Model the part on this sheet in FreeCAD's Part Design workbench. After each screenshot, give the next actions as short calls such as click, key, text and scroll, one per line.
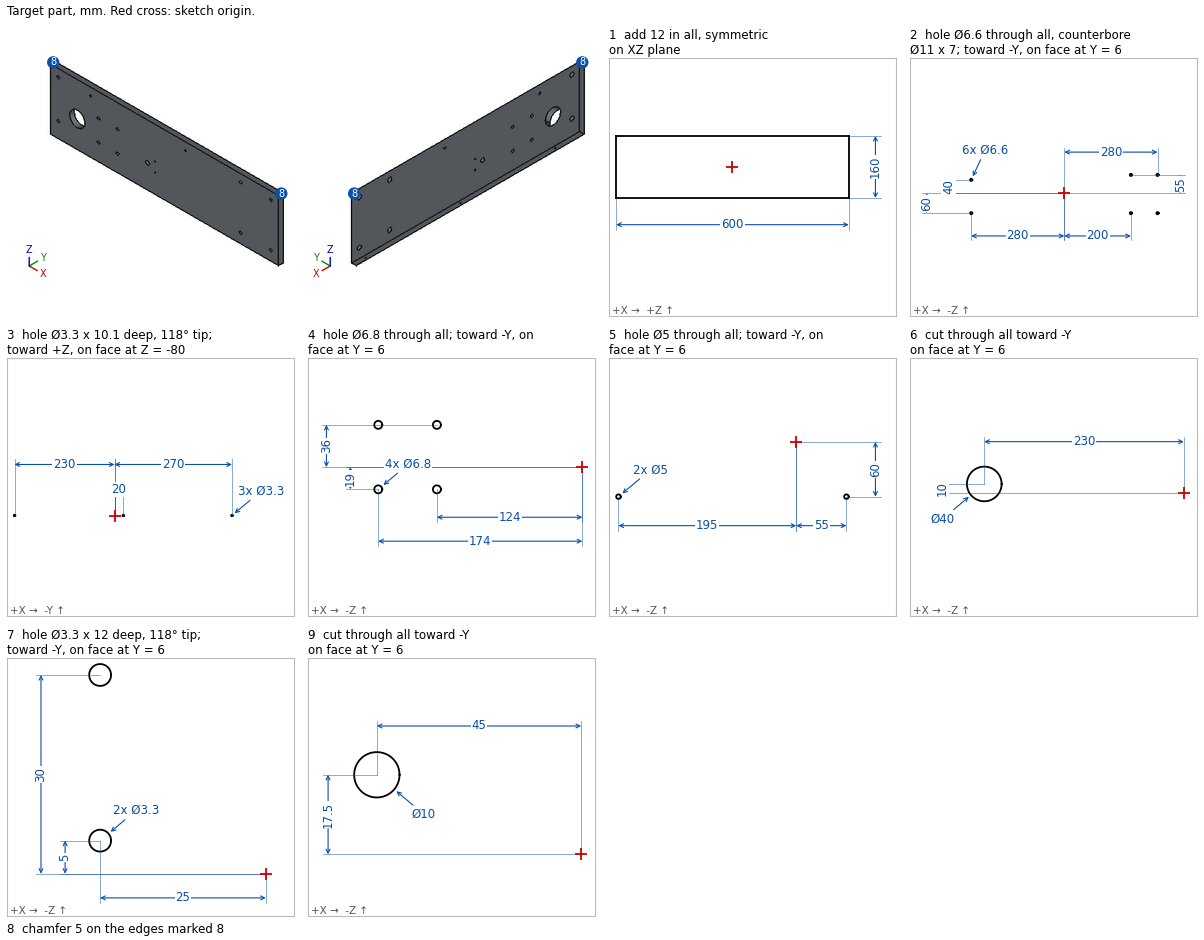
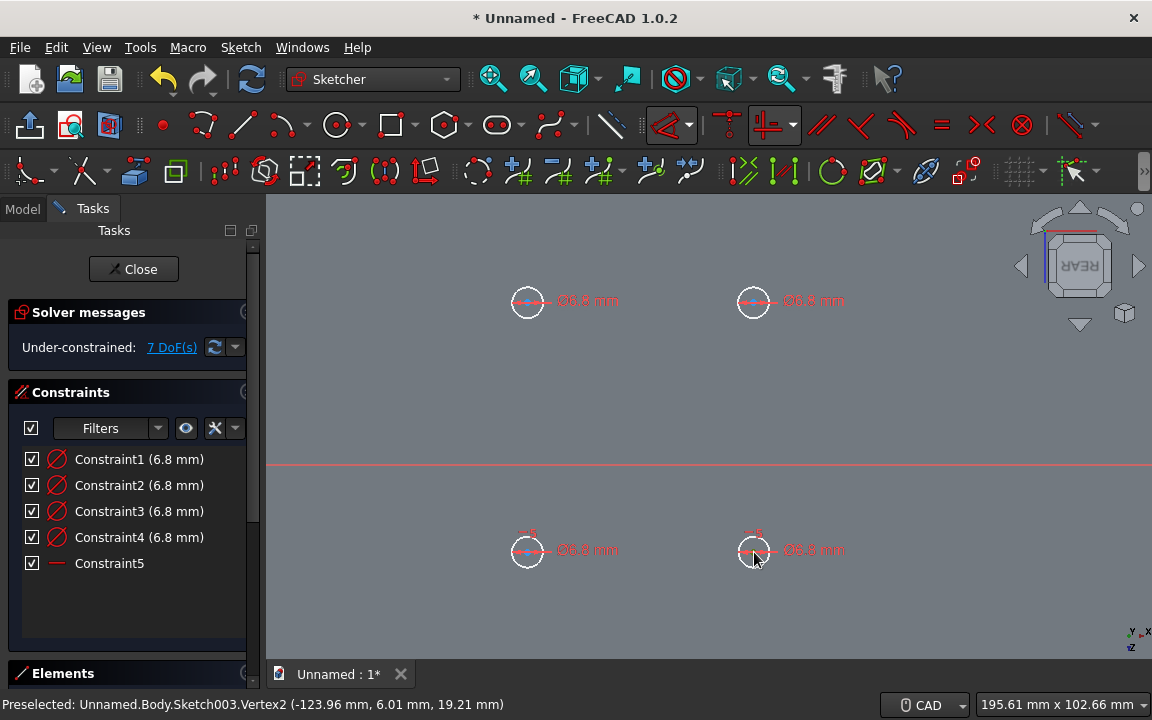
click(754, 303)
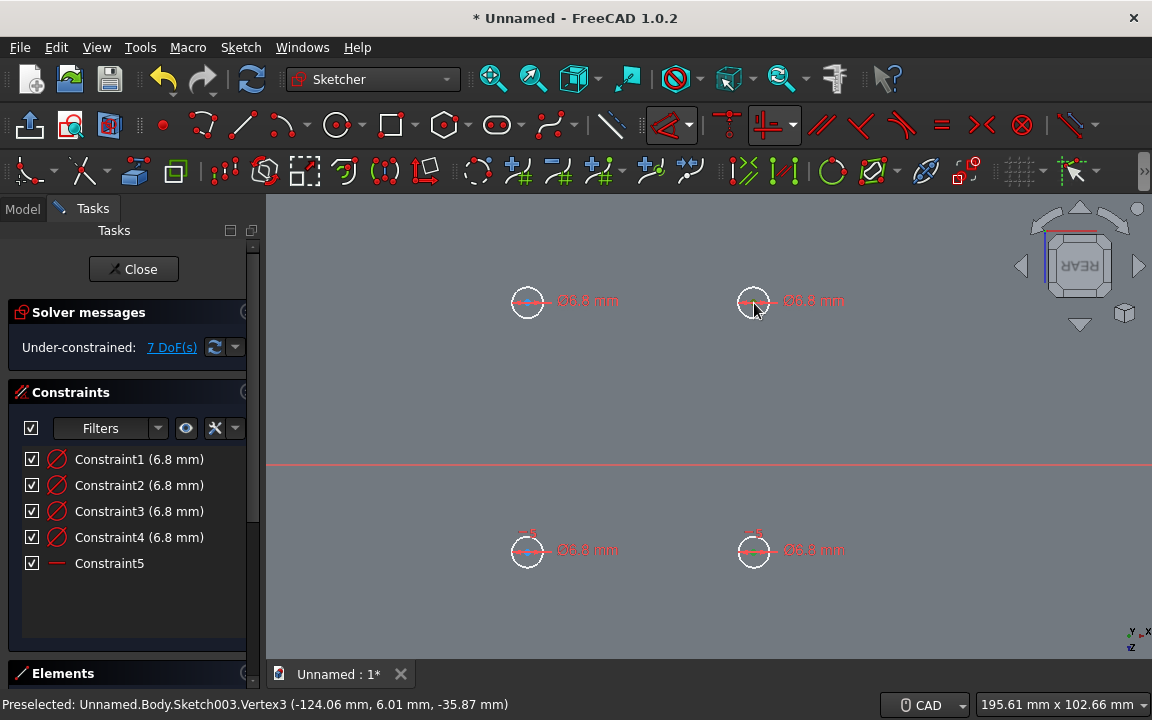
key(v)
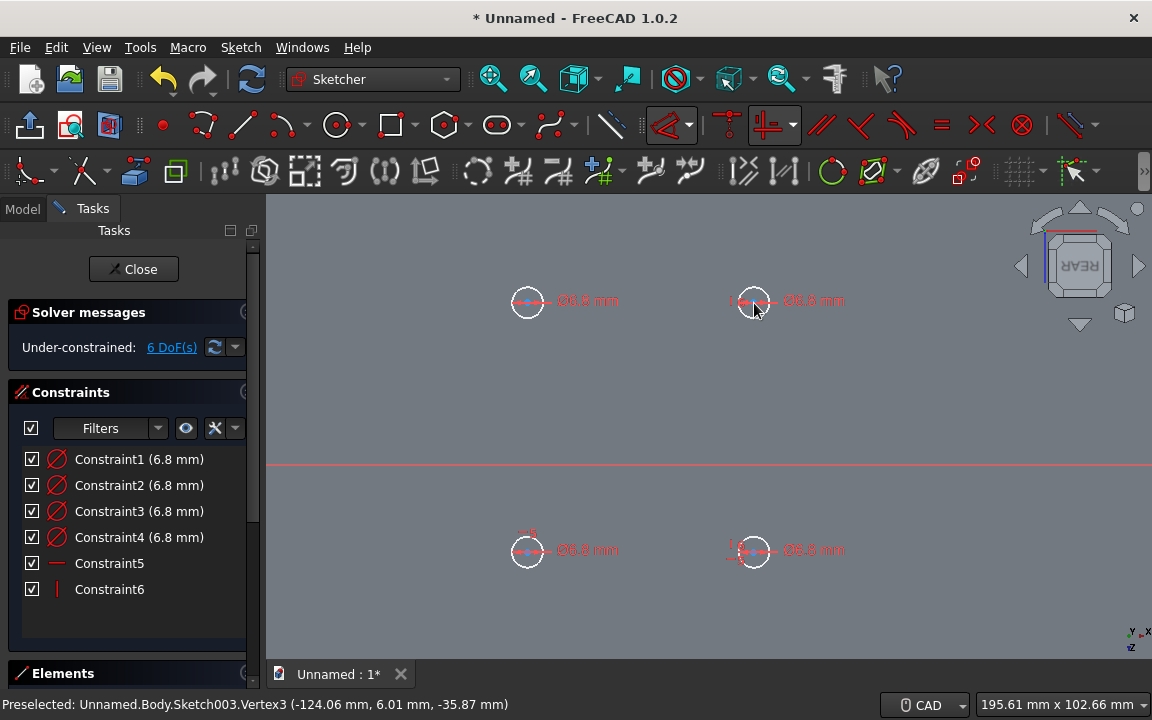
click(527, 552)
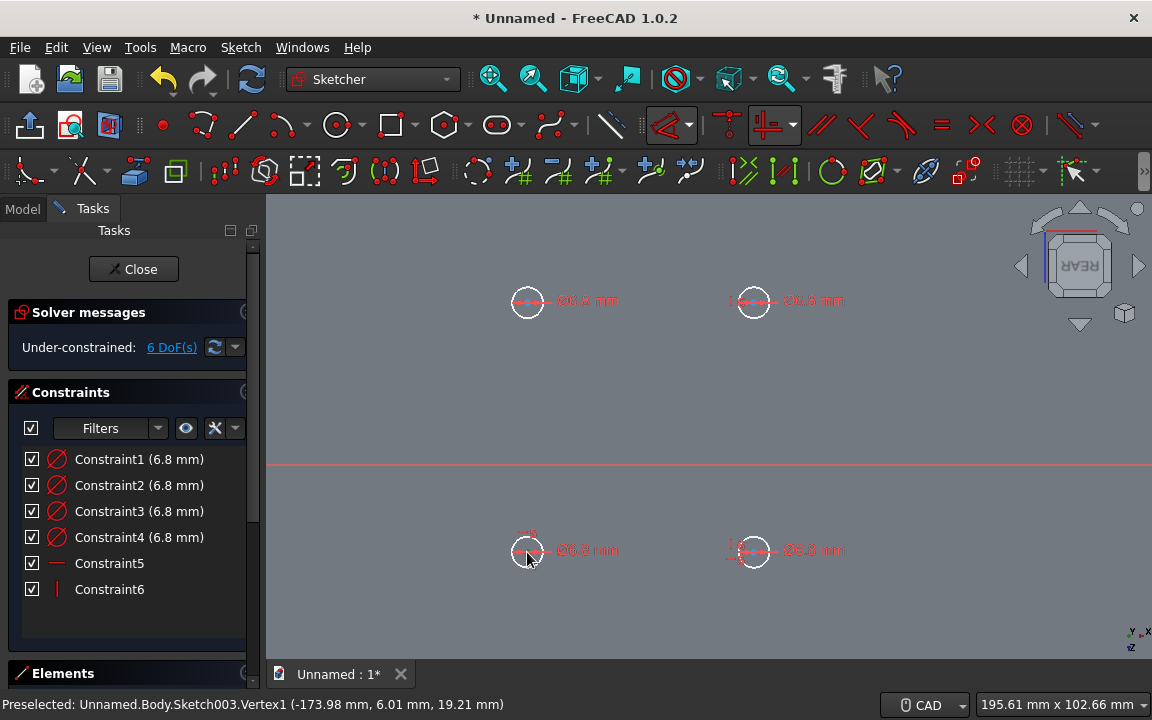
click(528, 303)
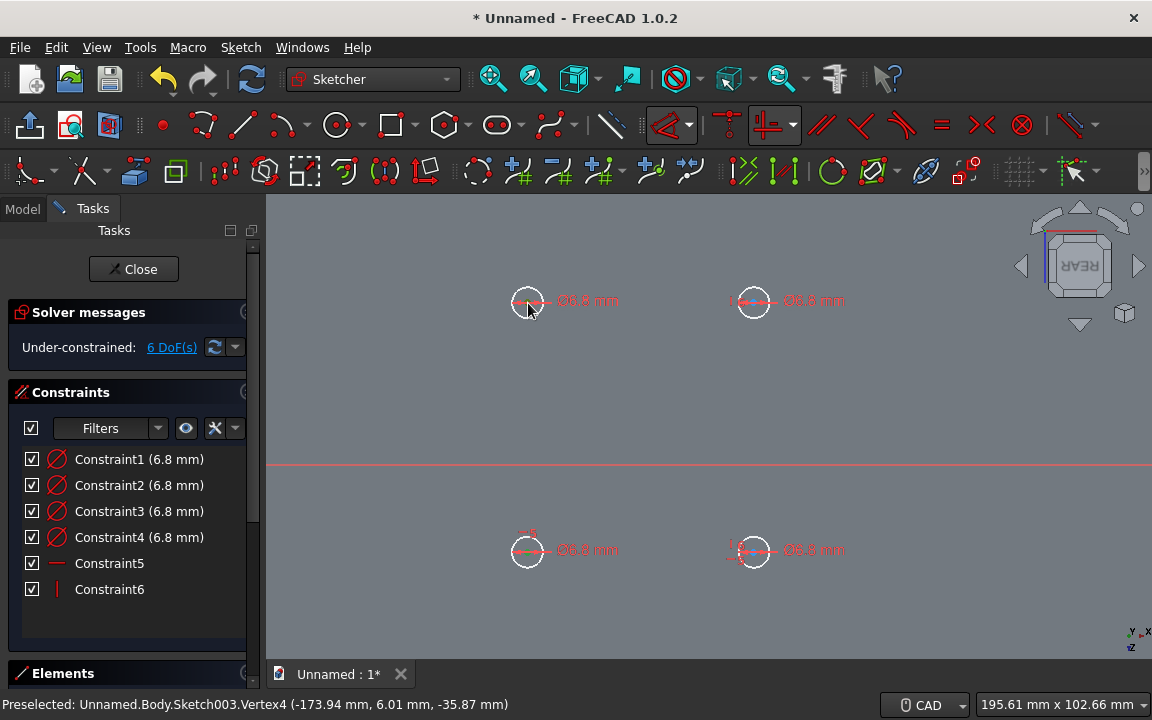
click(796, 126)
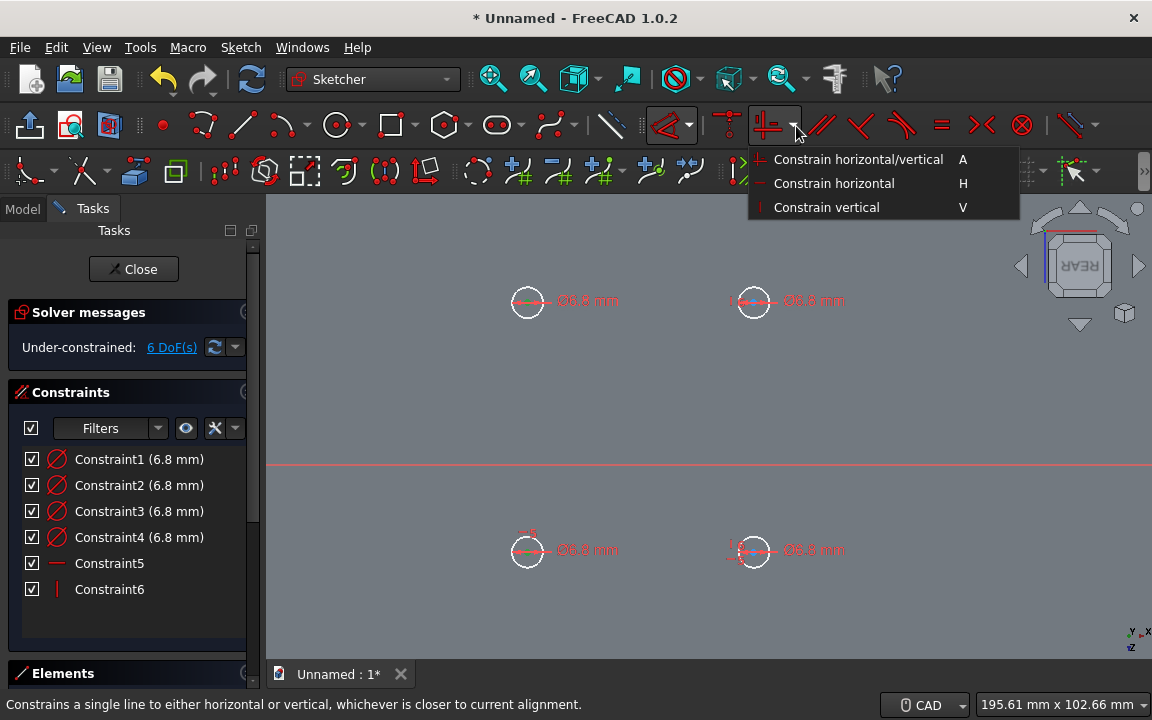
click(884, 207)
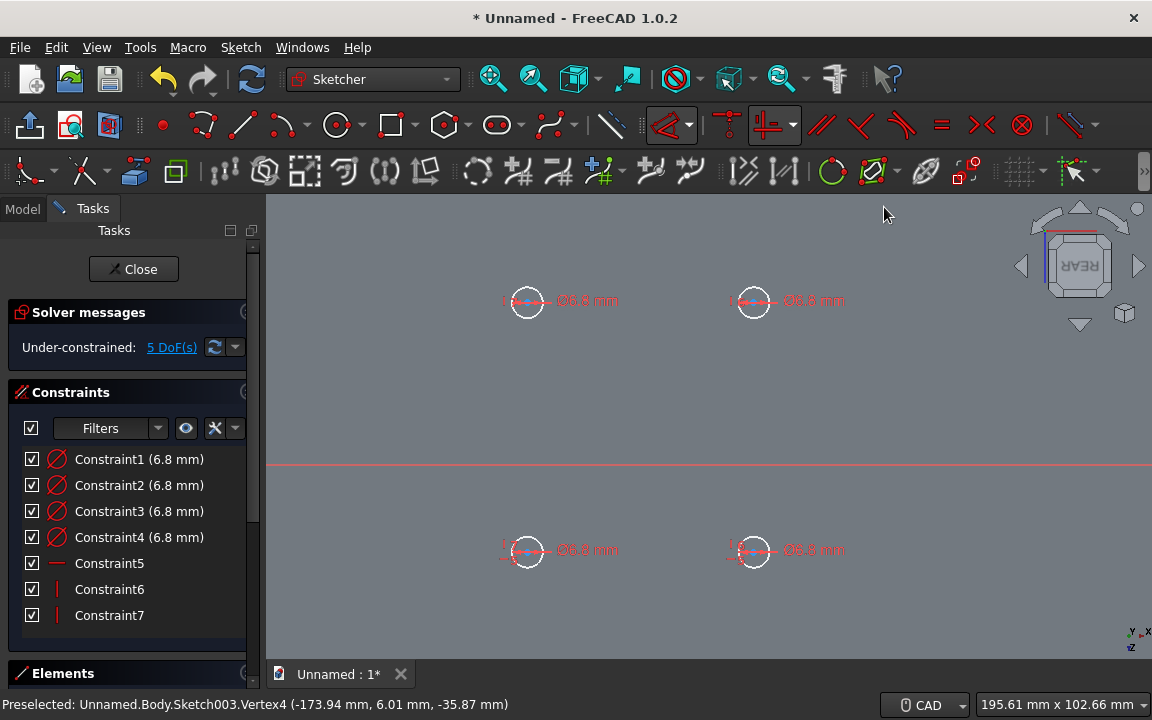
click(754, 303)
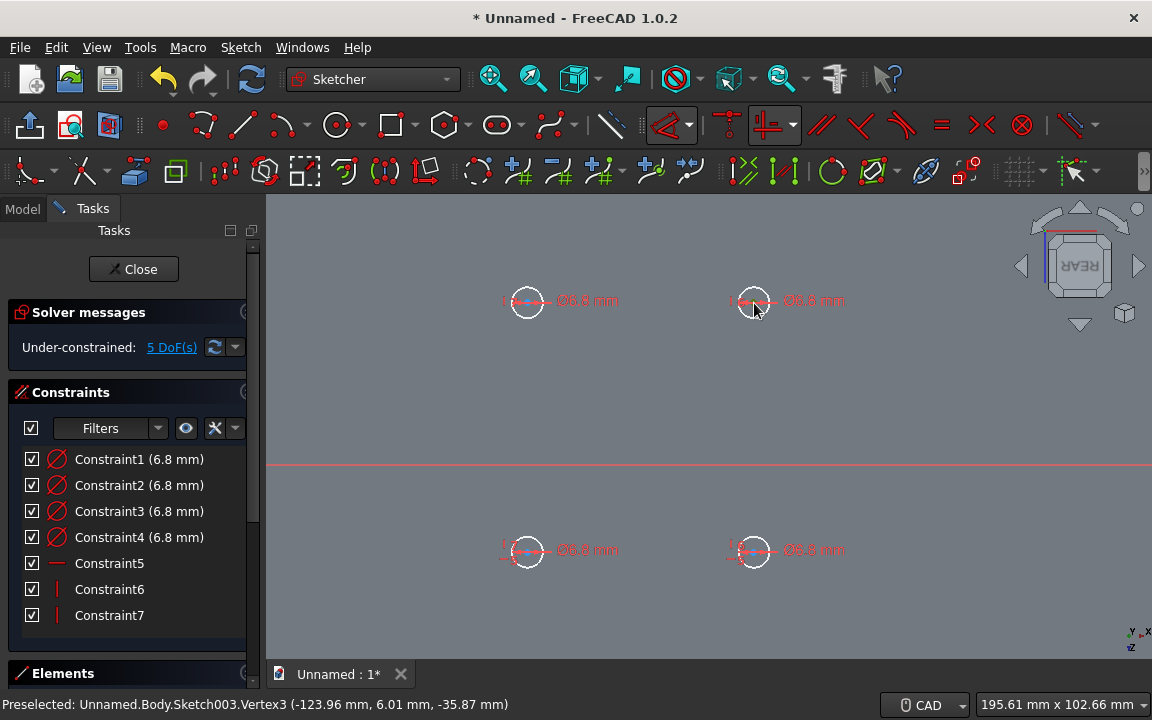
click(527, 303)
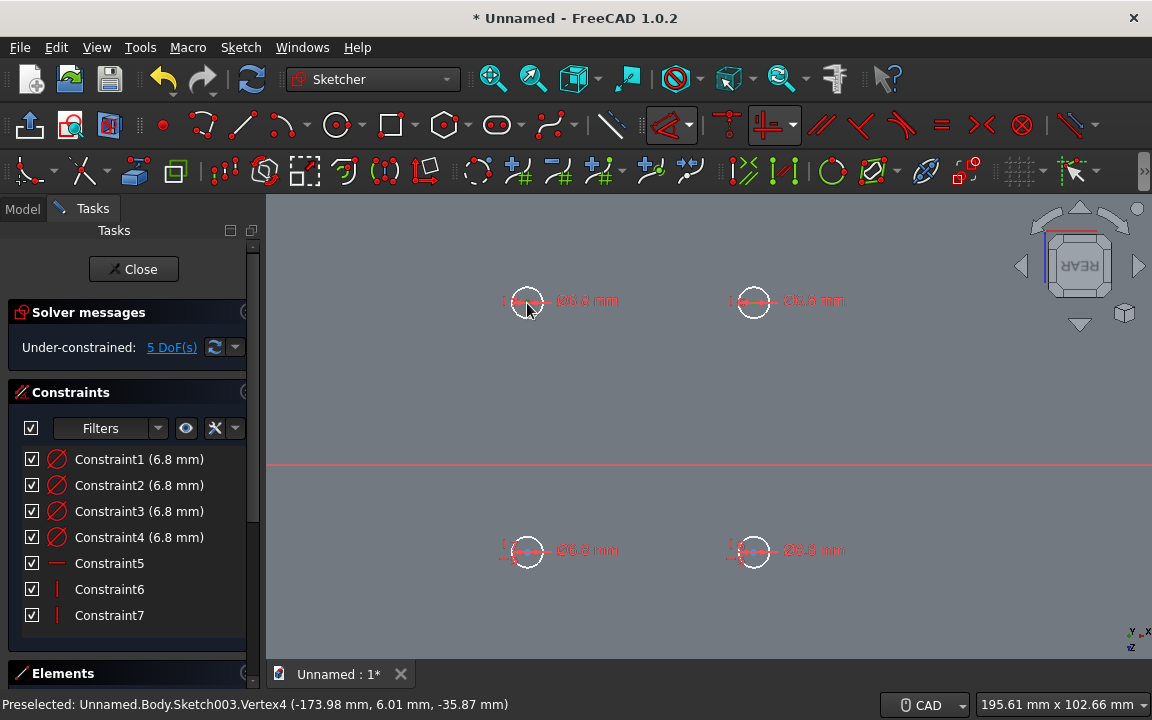
click(796, 126)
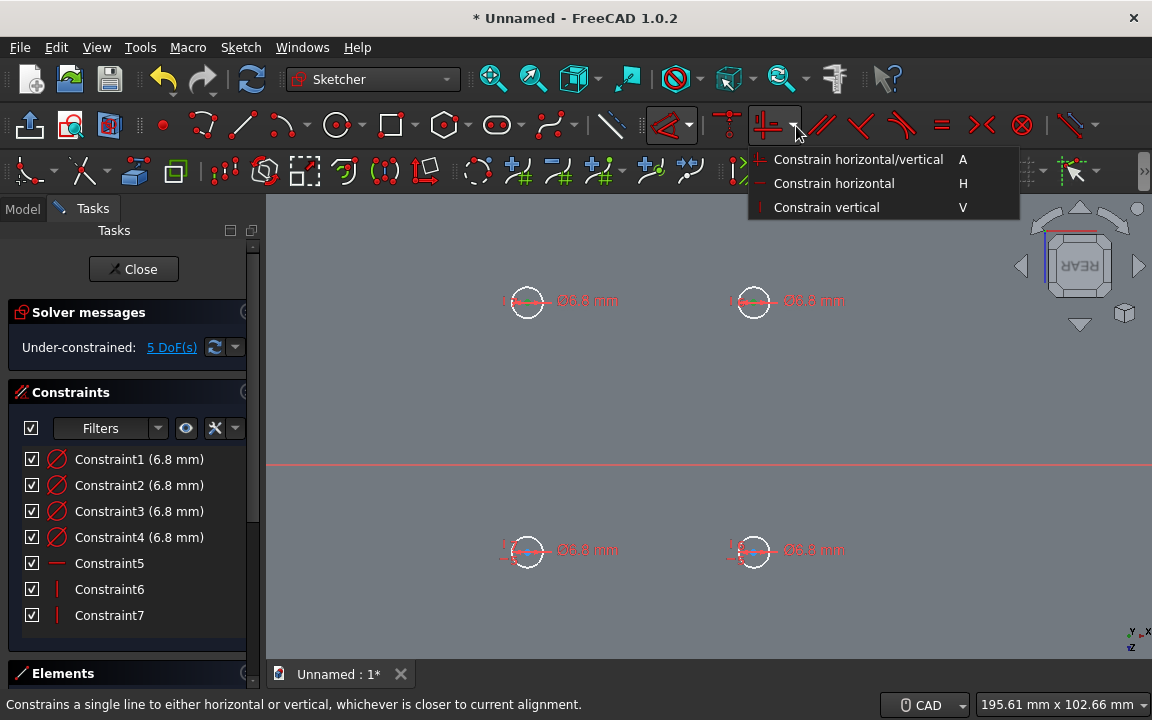
click(884, 183)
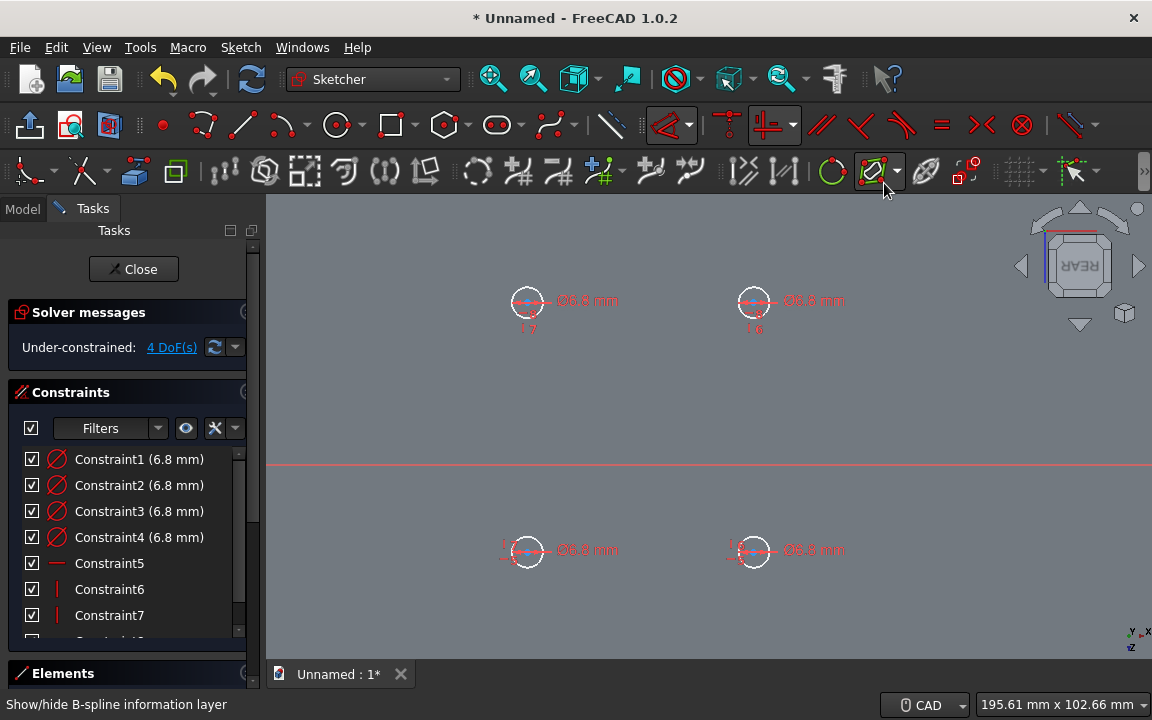
click(527, 552)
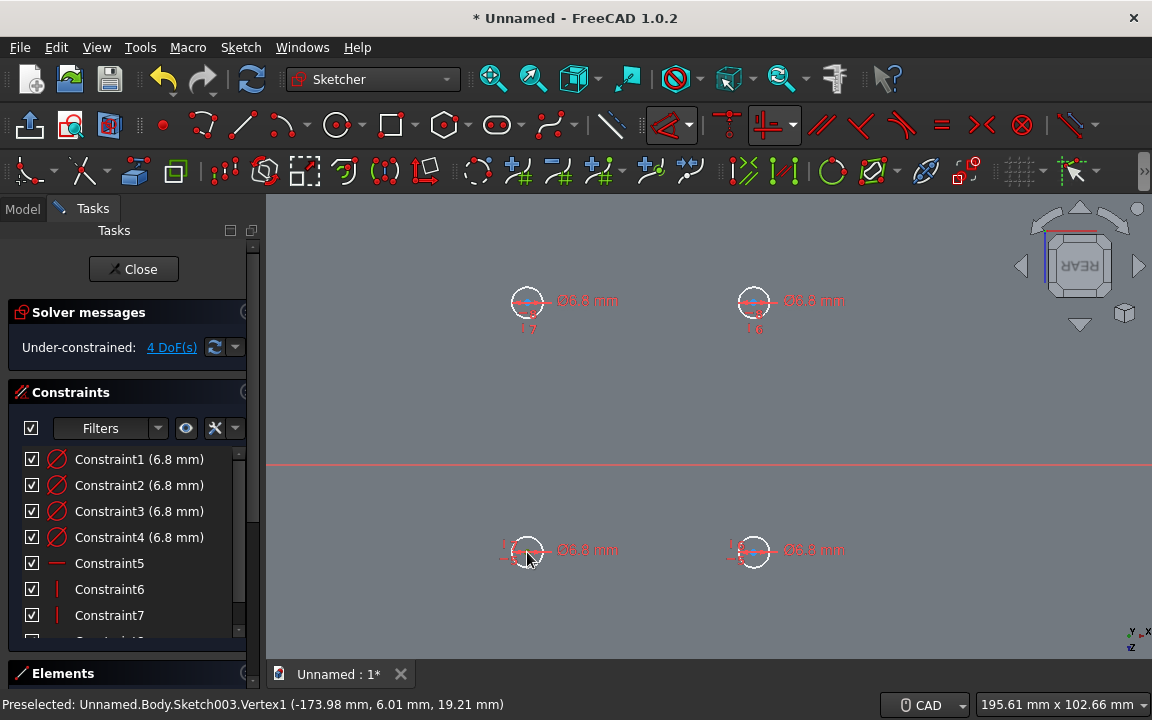
click(692, 126)